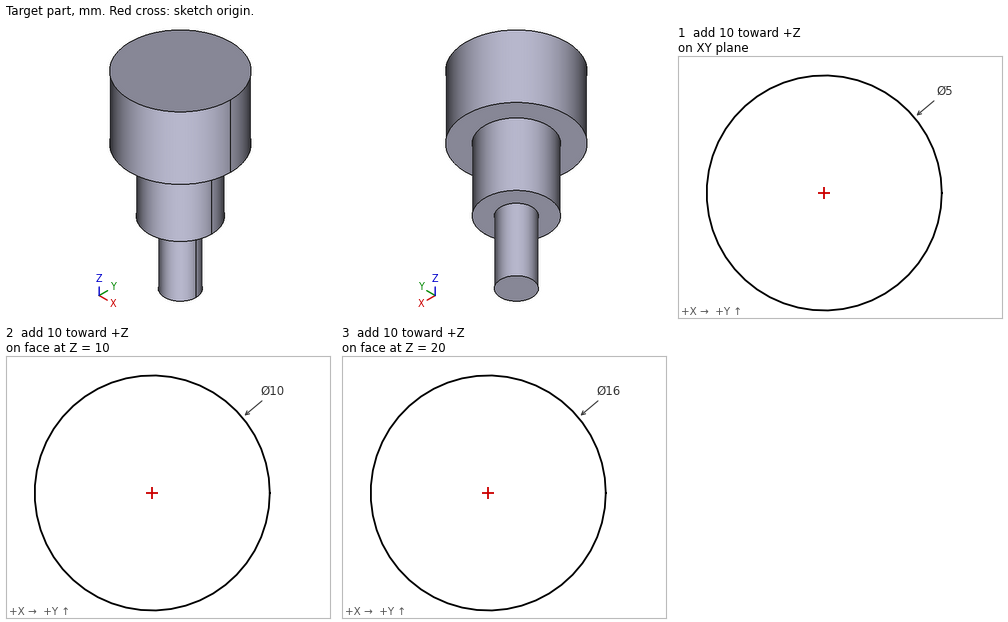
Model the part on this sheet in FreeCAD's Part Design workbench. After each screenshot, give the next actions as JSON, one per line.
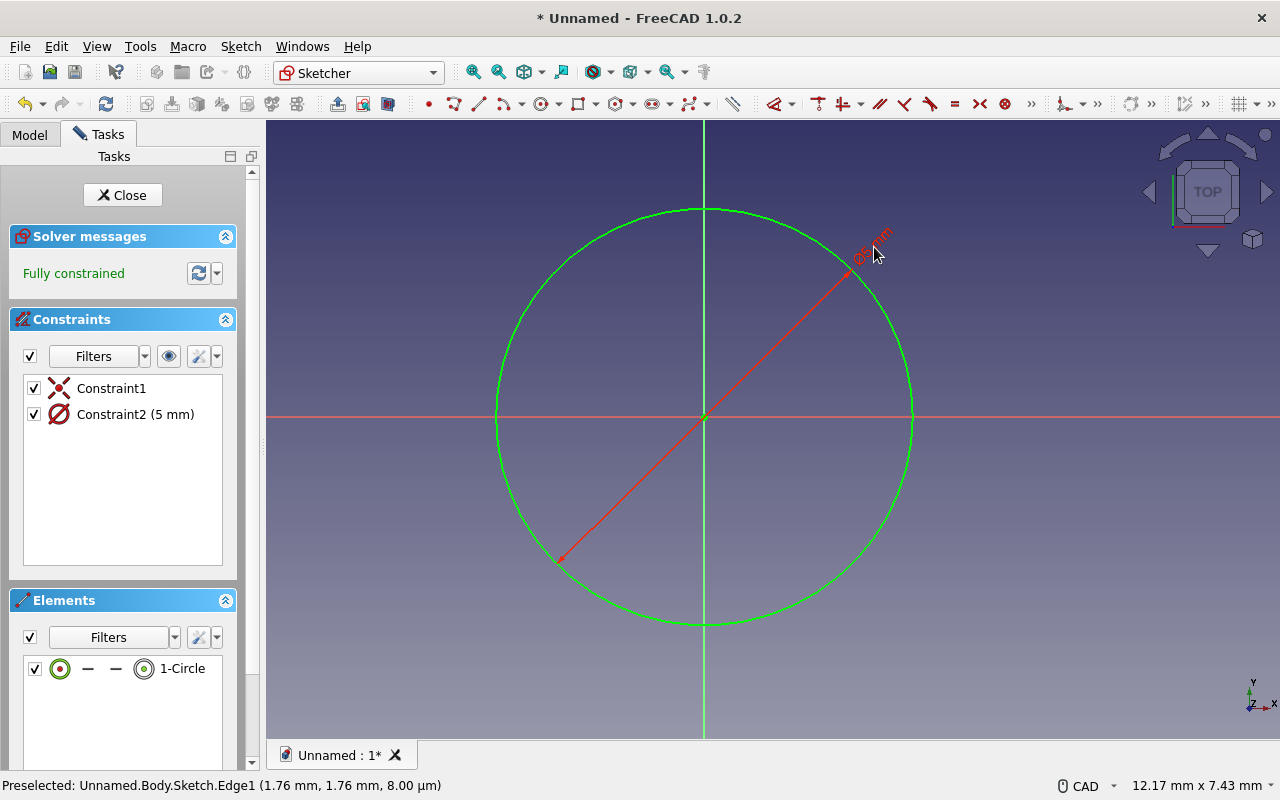
{"action": "left_click", "coordinate": [123, 195]}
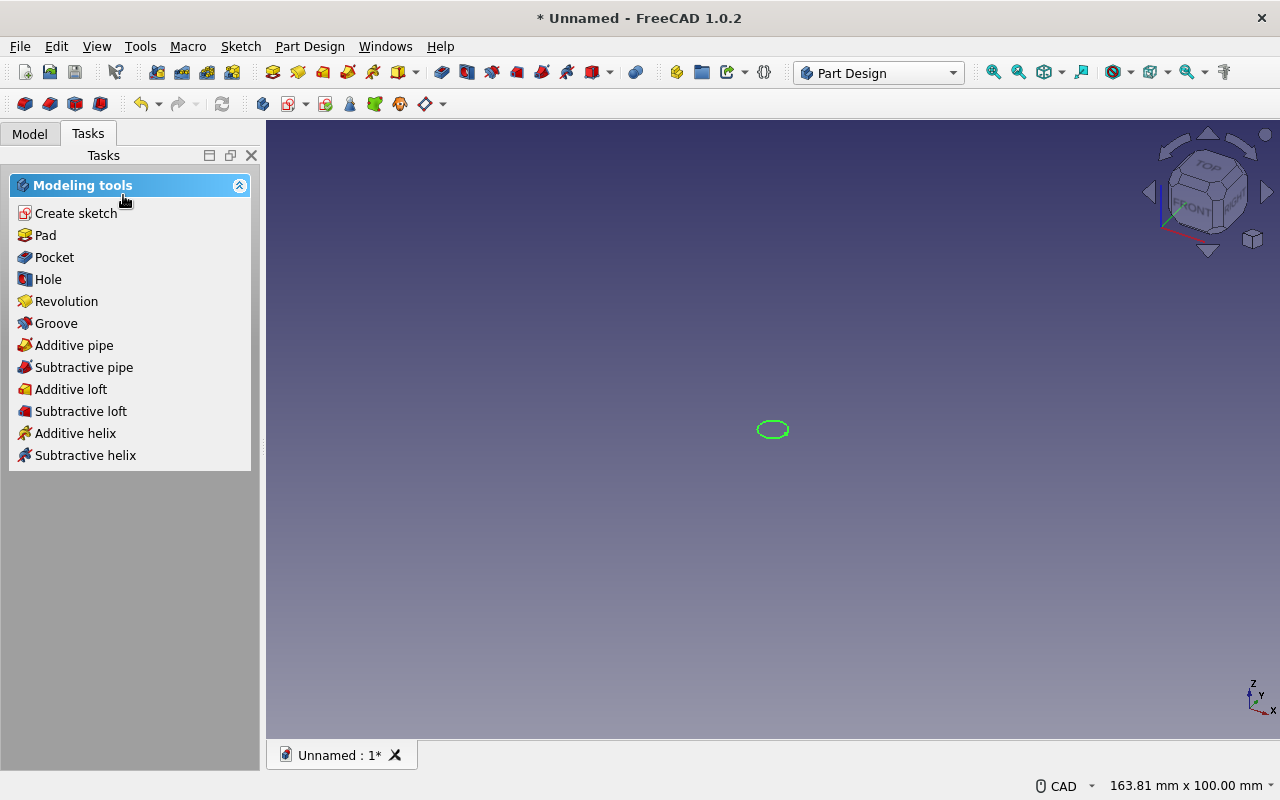
{"action": "left_click", "coordinate": [273, 72]}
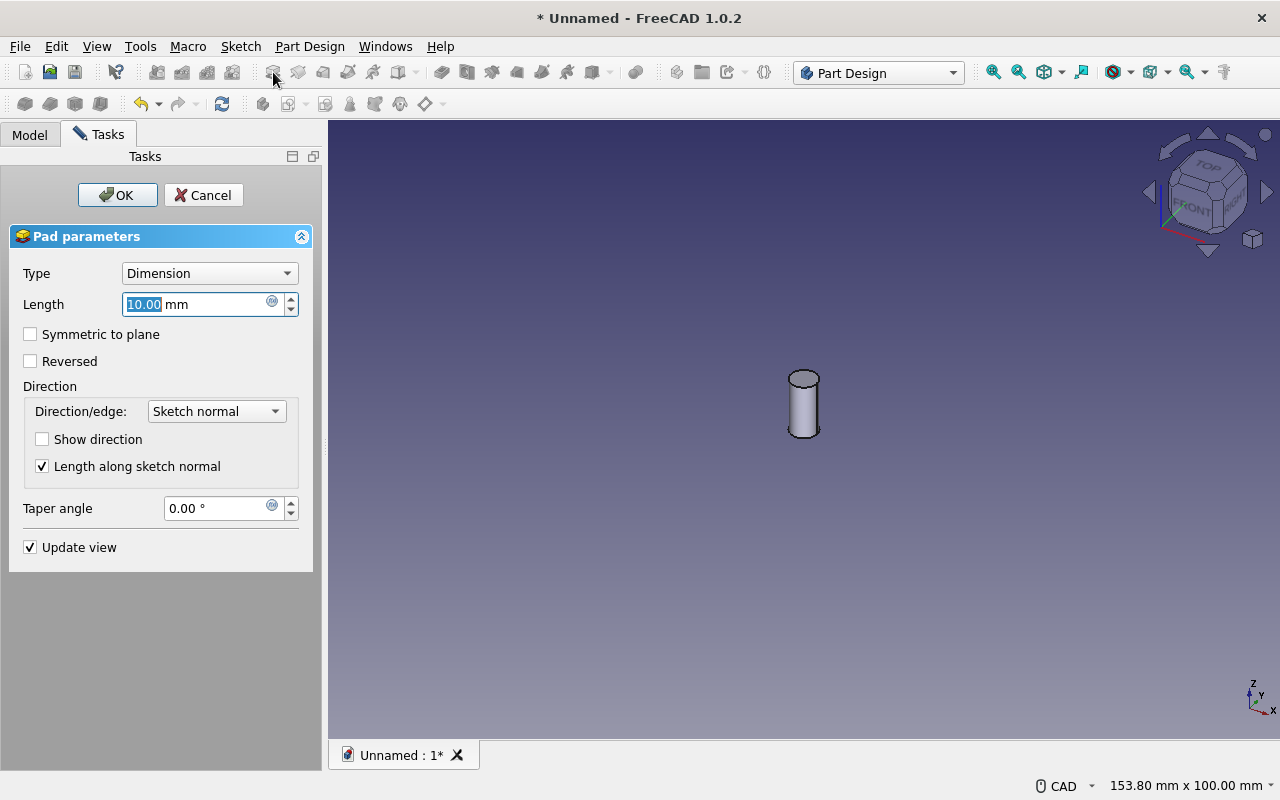
{"action": "type", "text": "10"}
{"action": "key", "text": "Tab"}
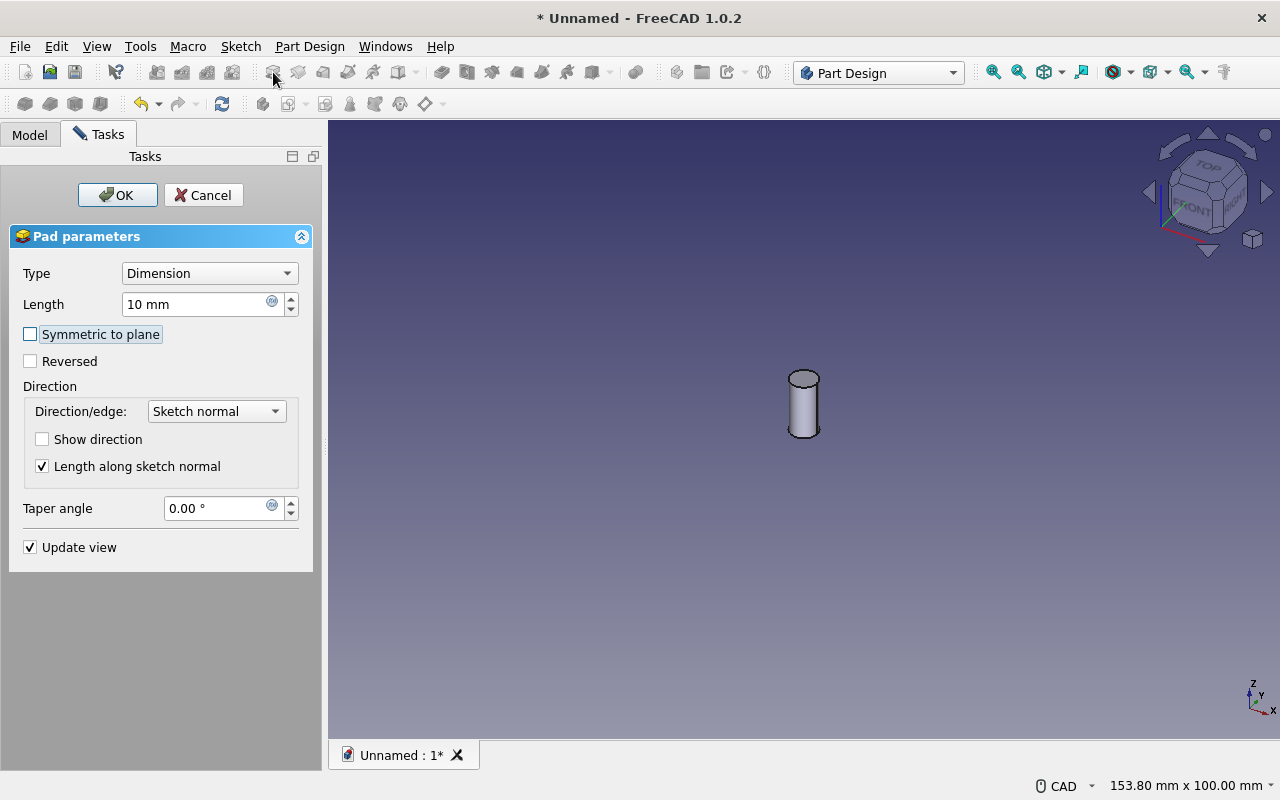
{"action": "left_click", "coordinate": [118, 195]}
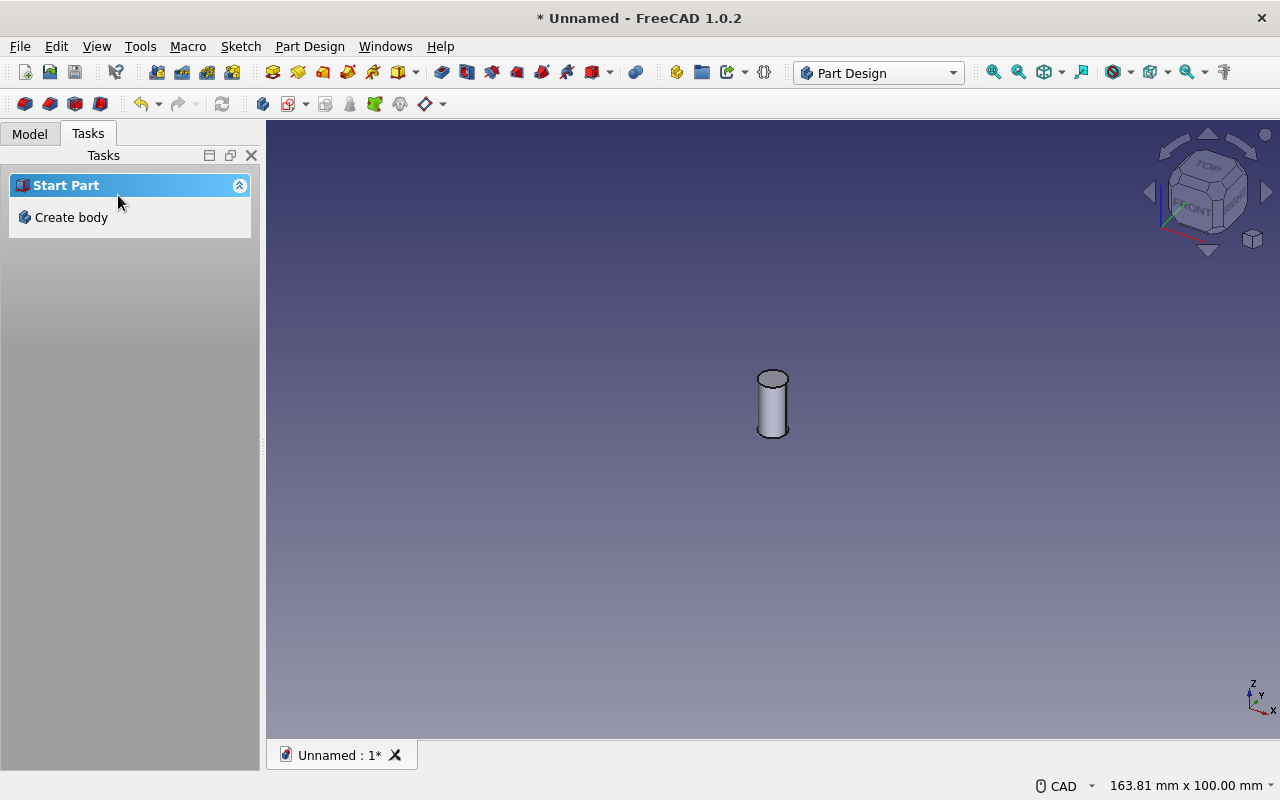
{"action": "key", "text": "v f"}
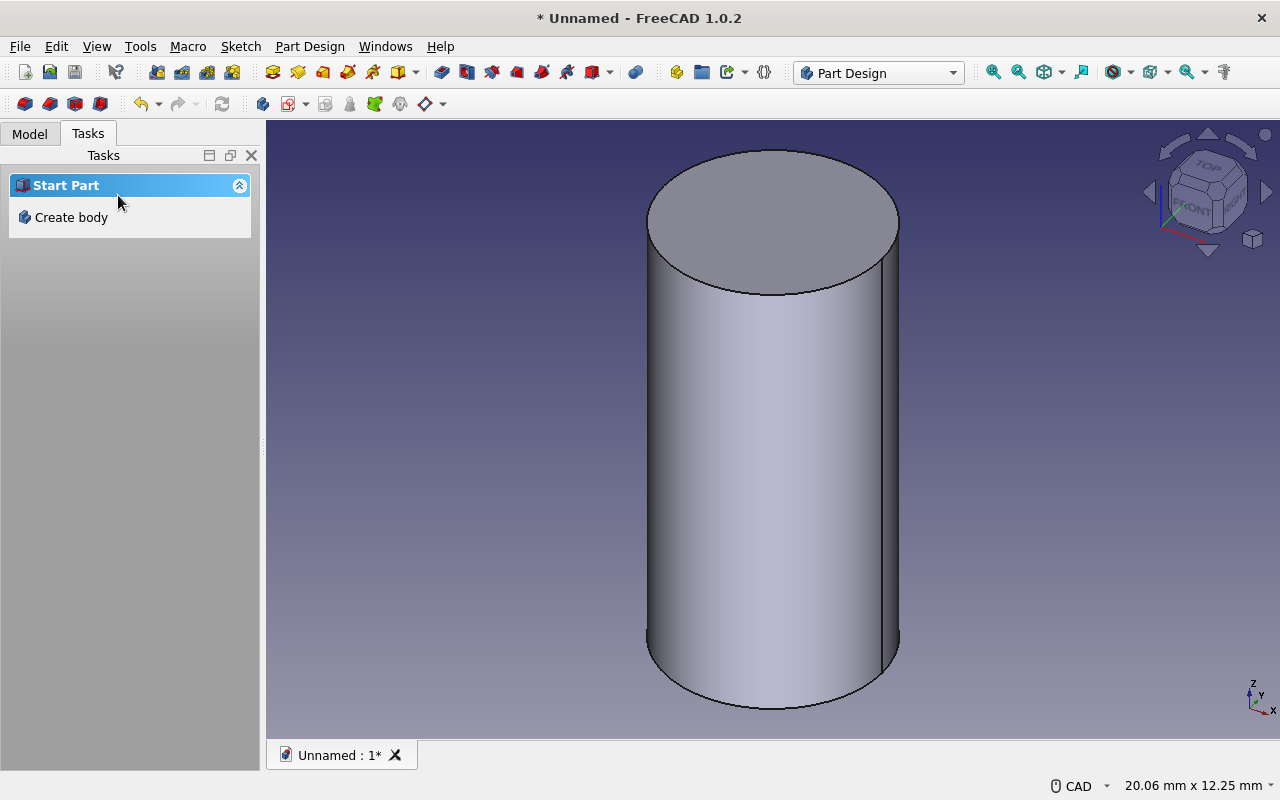
{"action": "left_click", "coordinate": [773, 221]}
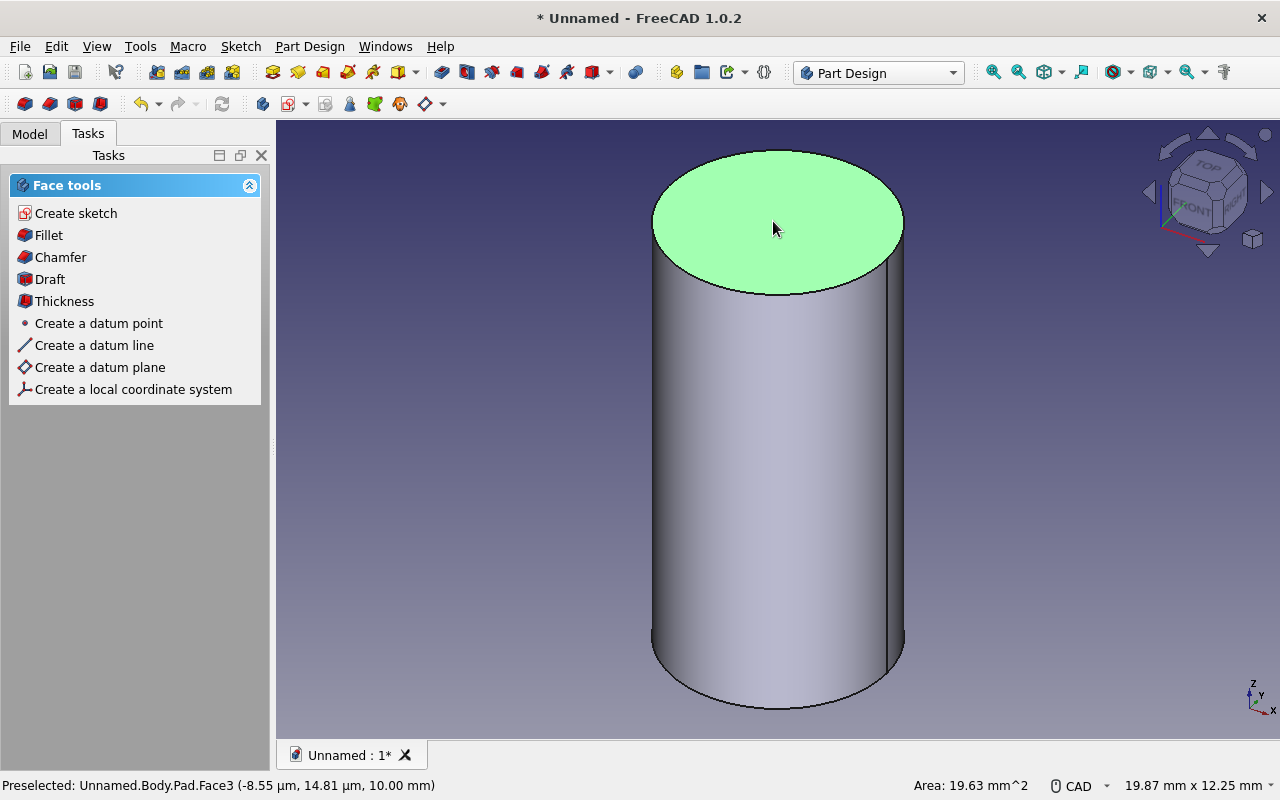
{"action": "left_click", "coordinate": [288, 104]}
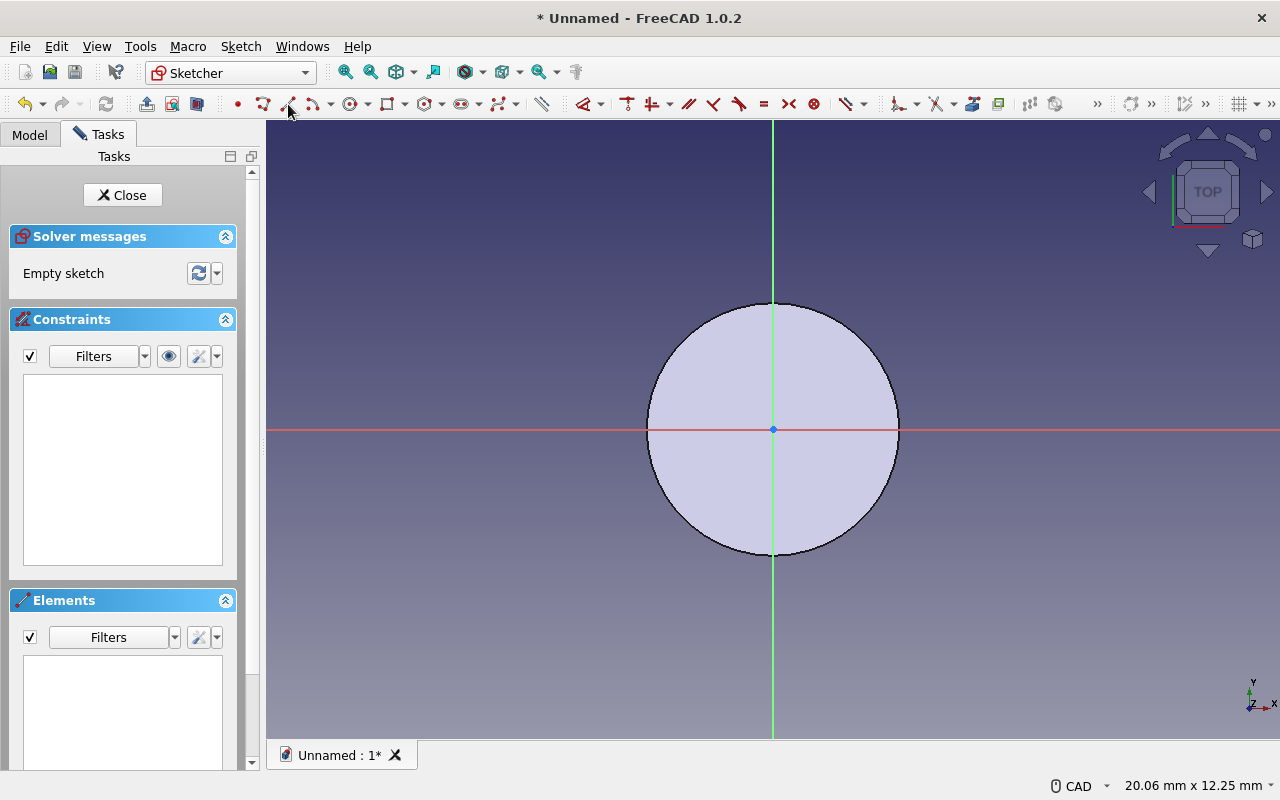
{"action": "left_click", "coordinate": [350, 104]}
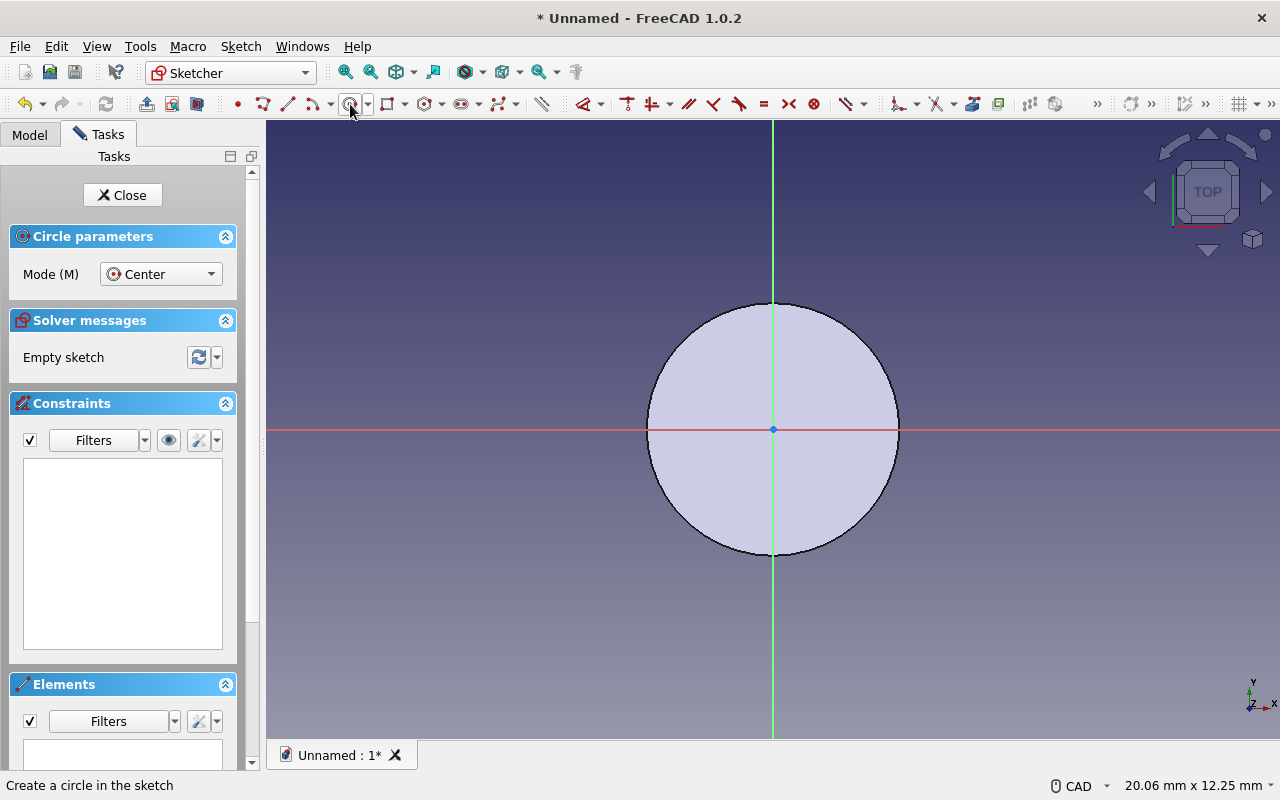
{"action": "left_click", "coordinate": [773, 430]}
{"action": "left_click", "coordinate": [952, 251]}
{"action": "key", "text": "Escape"}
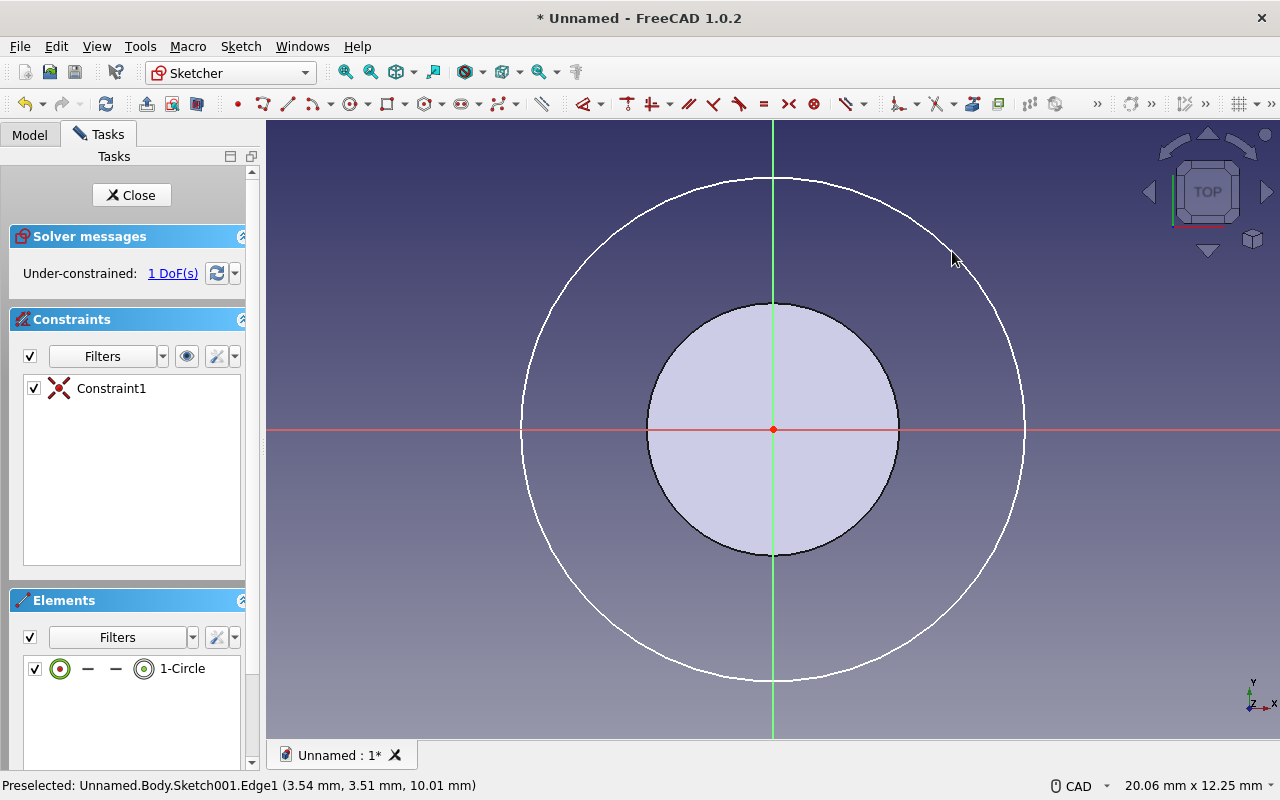
{"action": "key", "text": "d"}